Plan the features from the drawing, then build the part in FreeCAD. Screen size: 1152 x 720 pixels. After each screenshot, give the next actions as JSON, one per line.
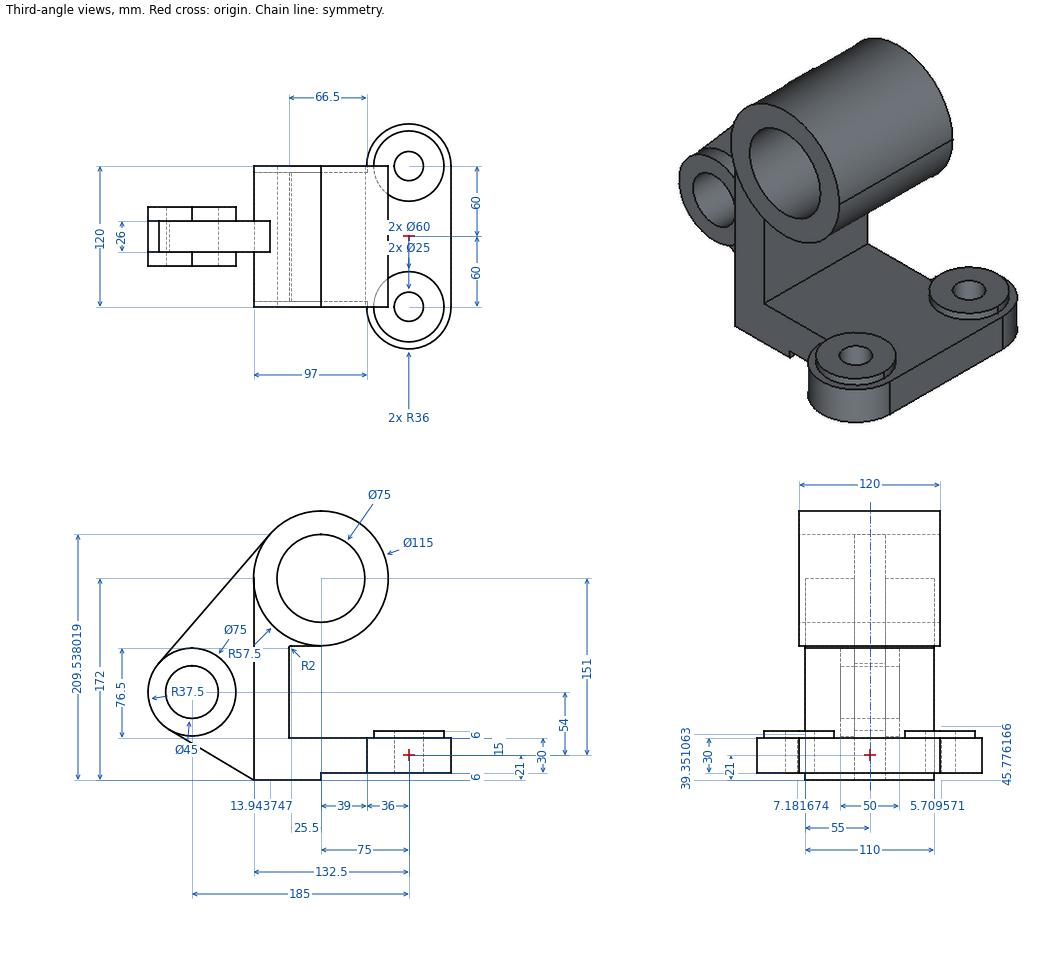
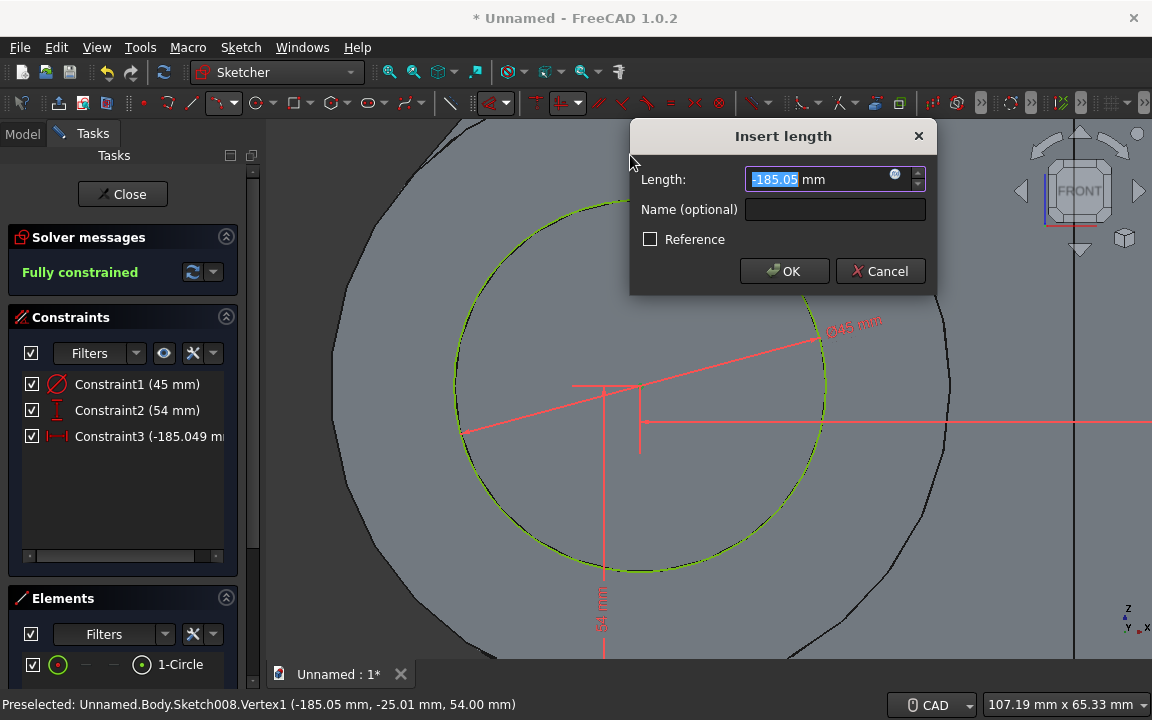
{"action": "type", "text": "-185"}
{"action": "key", "text": "Return"}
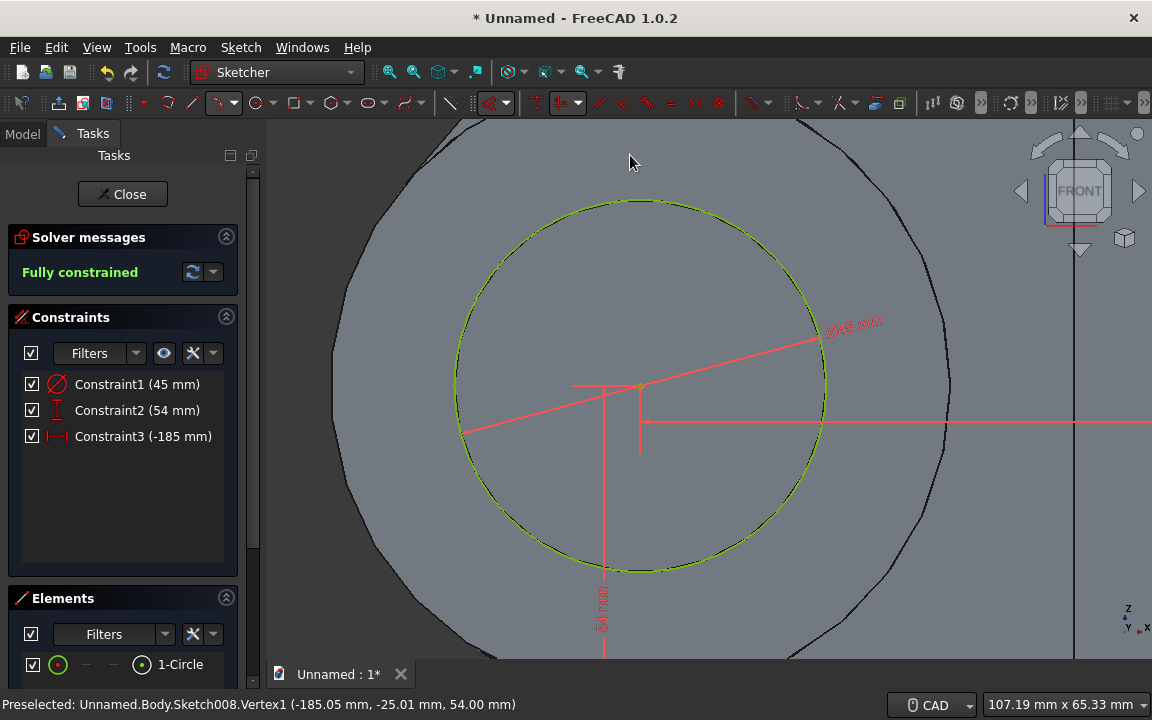
{"action": "left_click", "coordinate": [123, 194]}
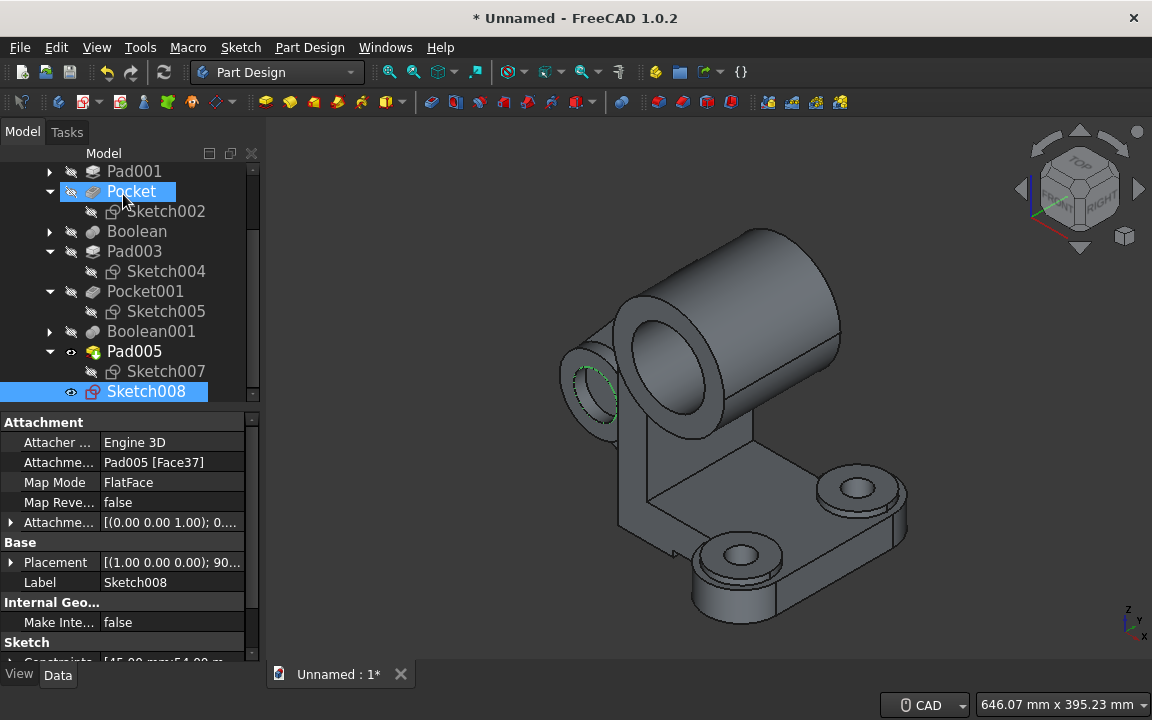
{"action": "left_click", "coordinate": [432, 102]}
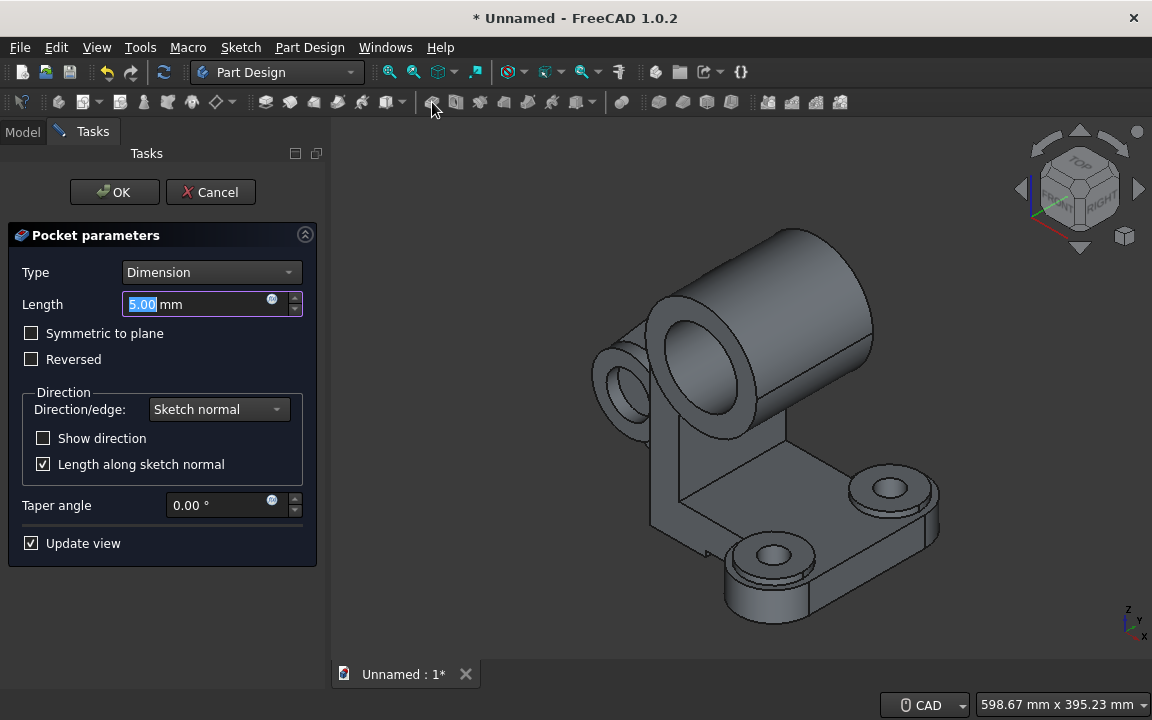
{"action": "left_click", "coordinate": [212, 272]}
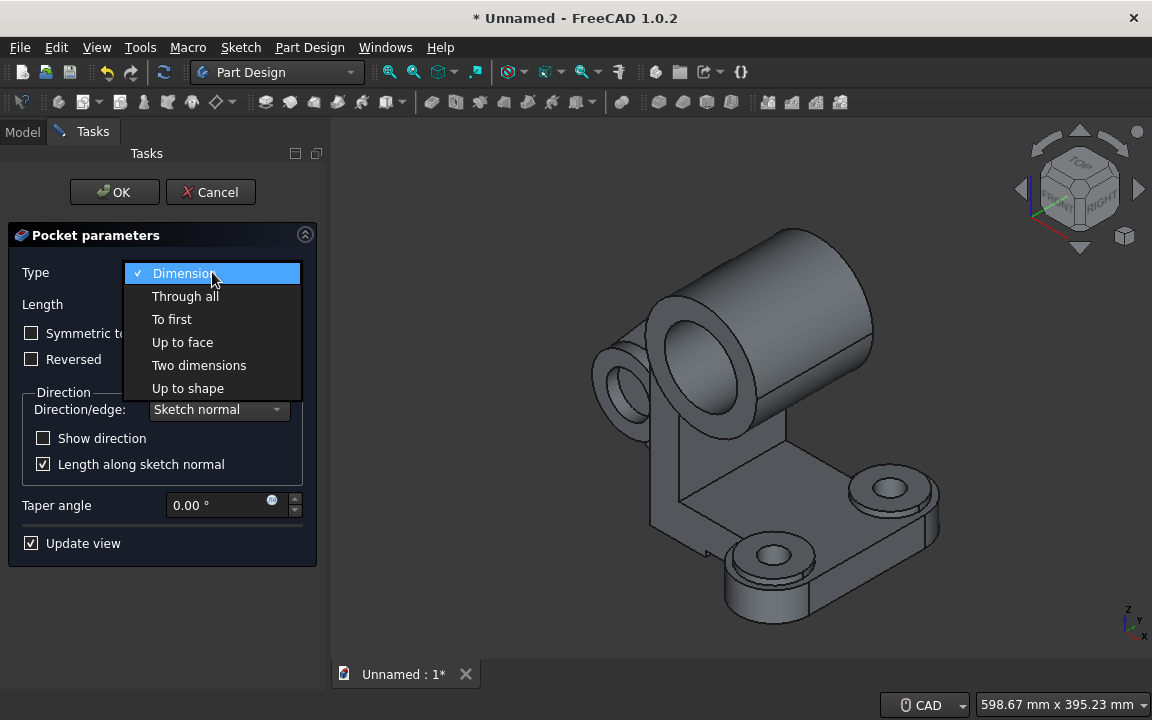
{"action": "left_click", "coordinate": [212, 296]}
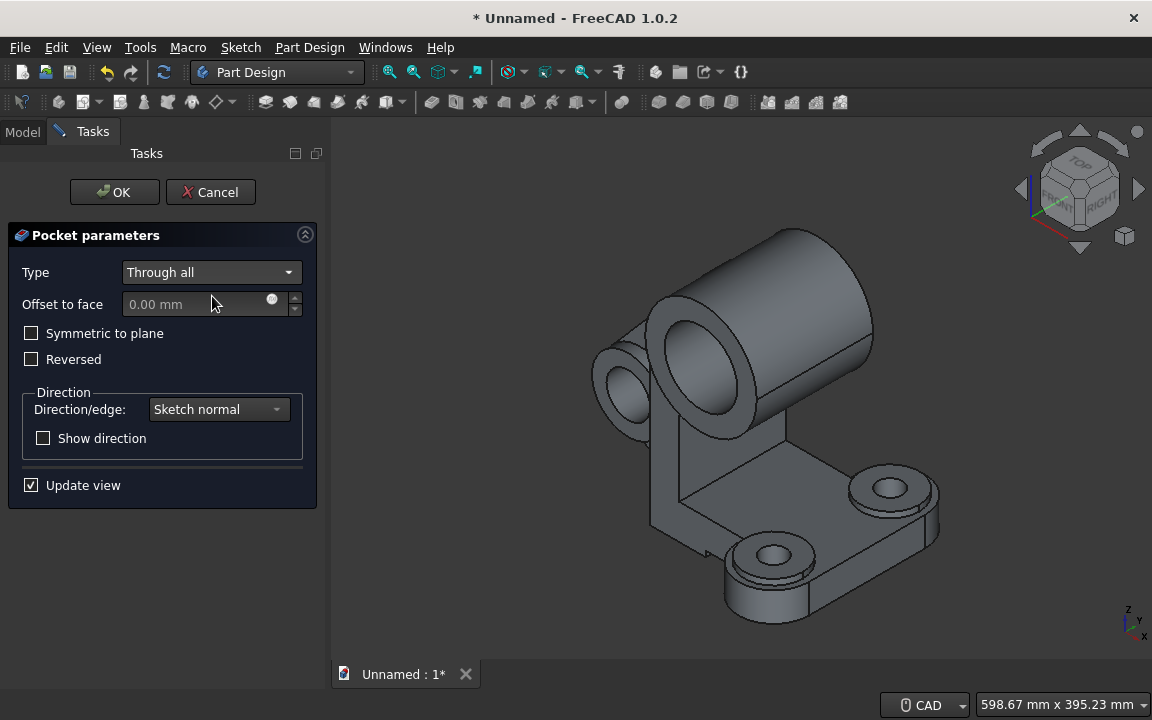
{"action": "left_click", "coordinate": [115, 192]}